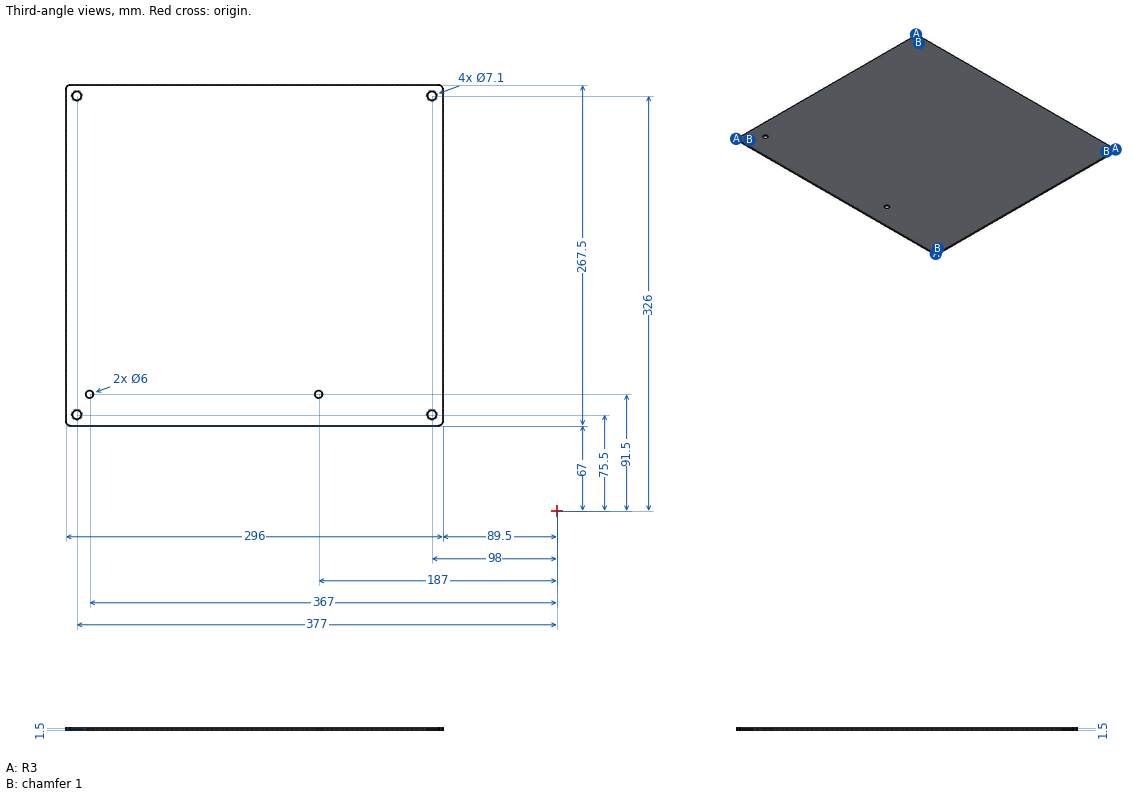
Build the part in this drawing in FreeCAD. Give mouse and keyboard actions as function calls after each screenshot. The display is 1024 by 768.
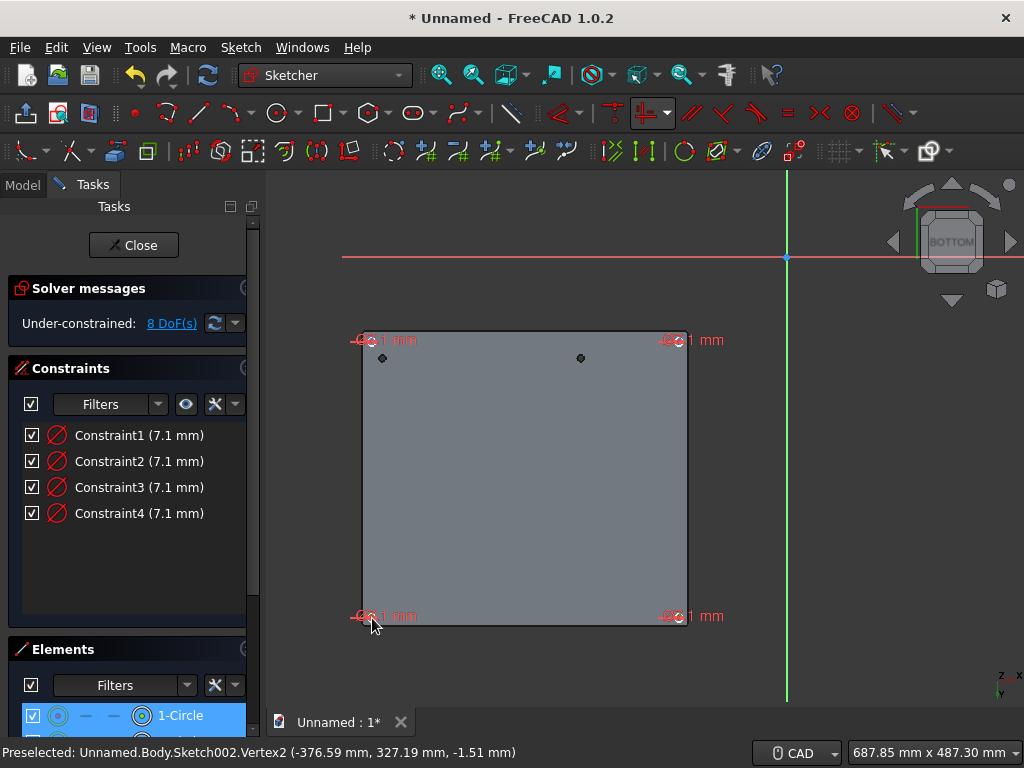
click(670, 114)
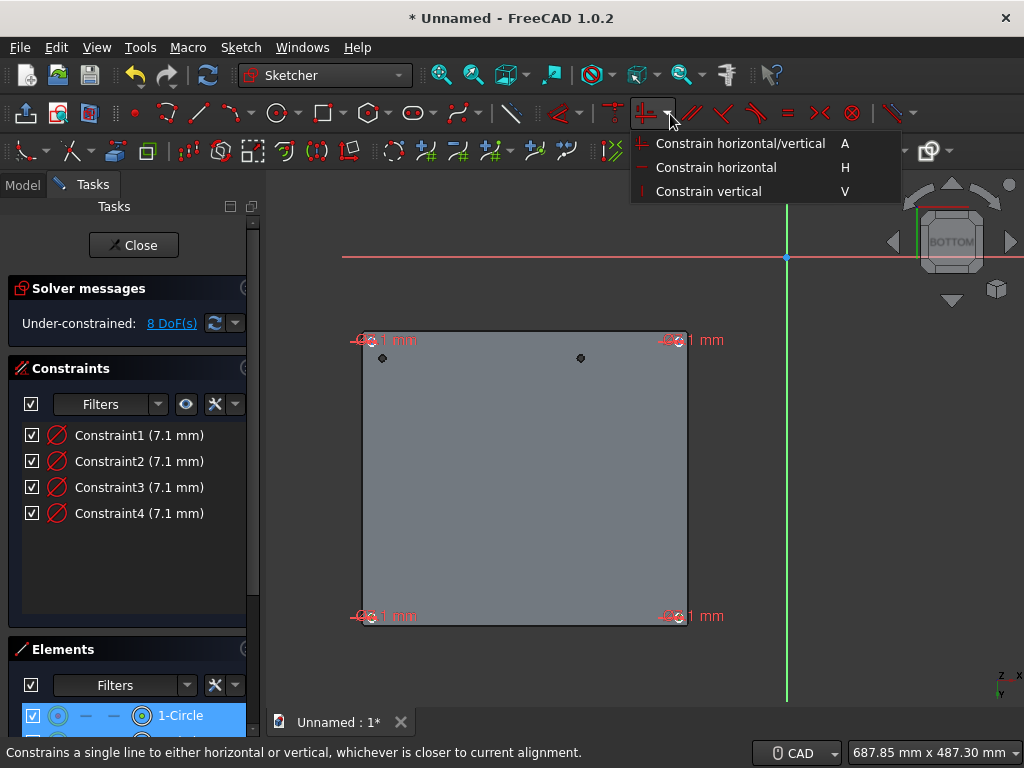
click(766, 167)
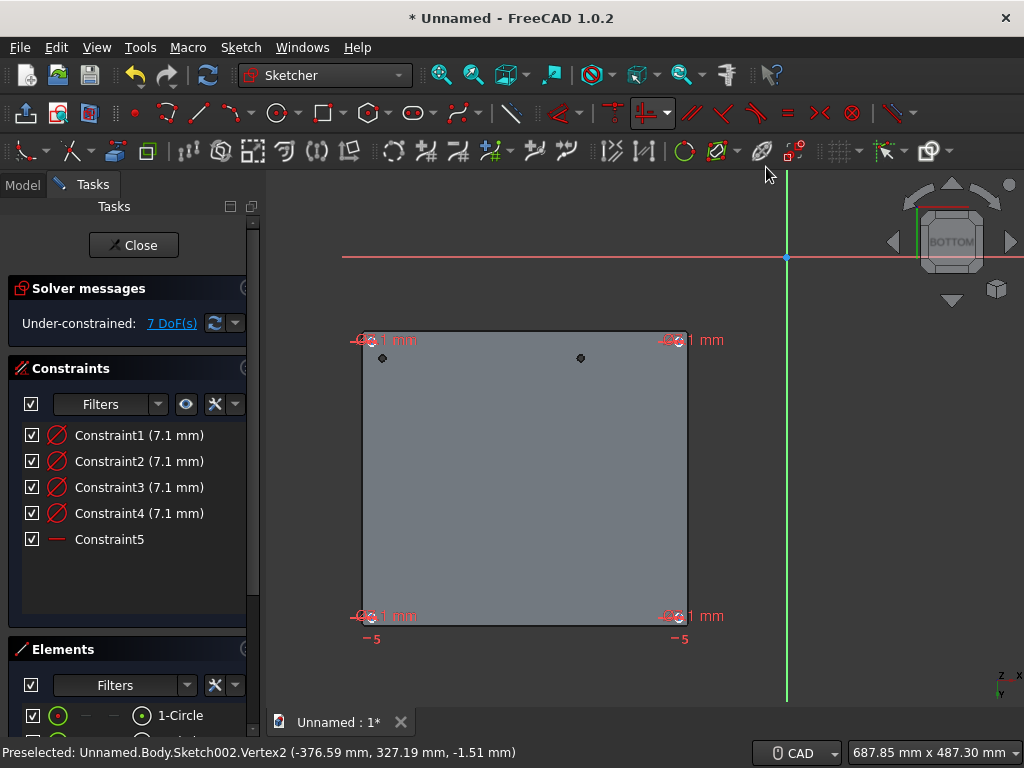
click(372, 618)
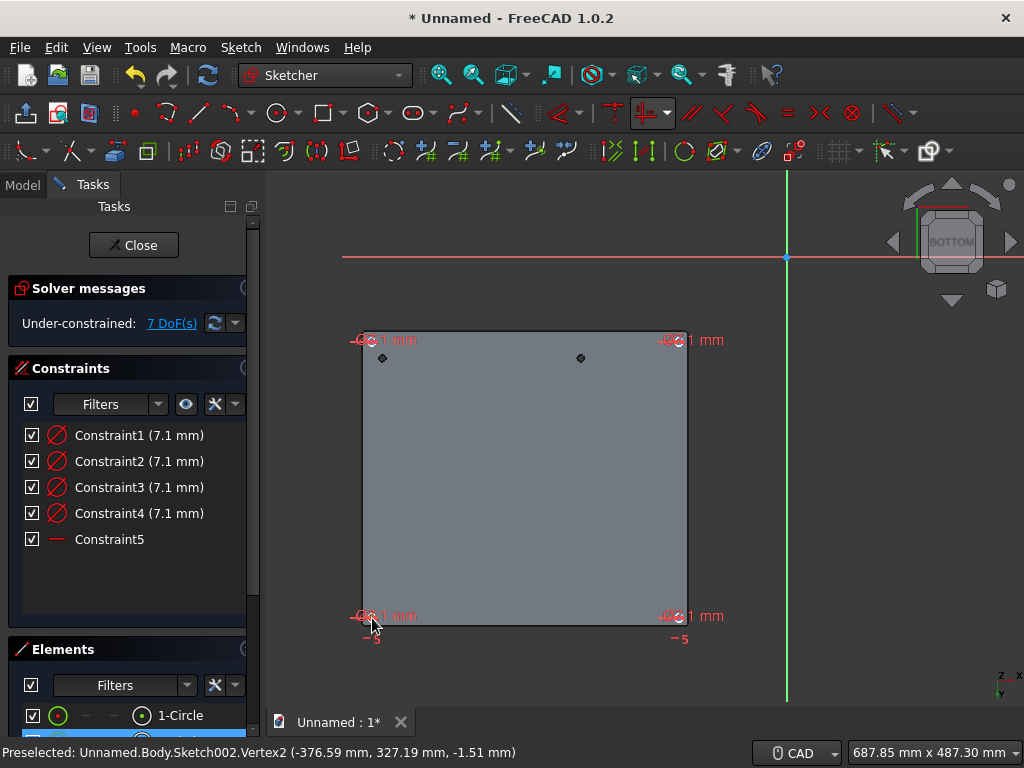
click(372, 342)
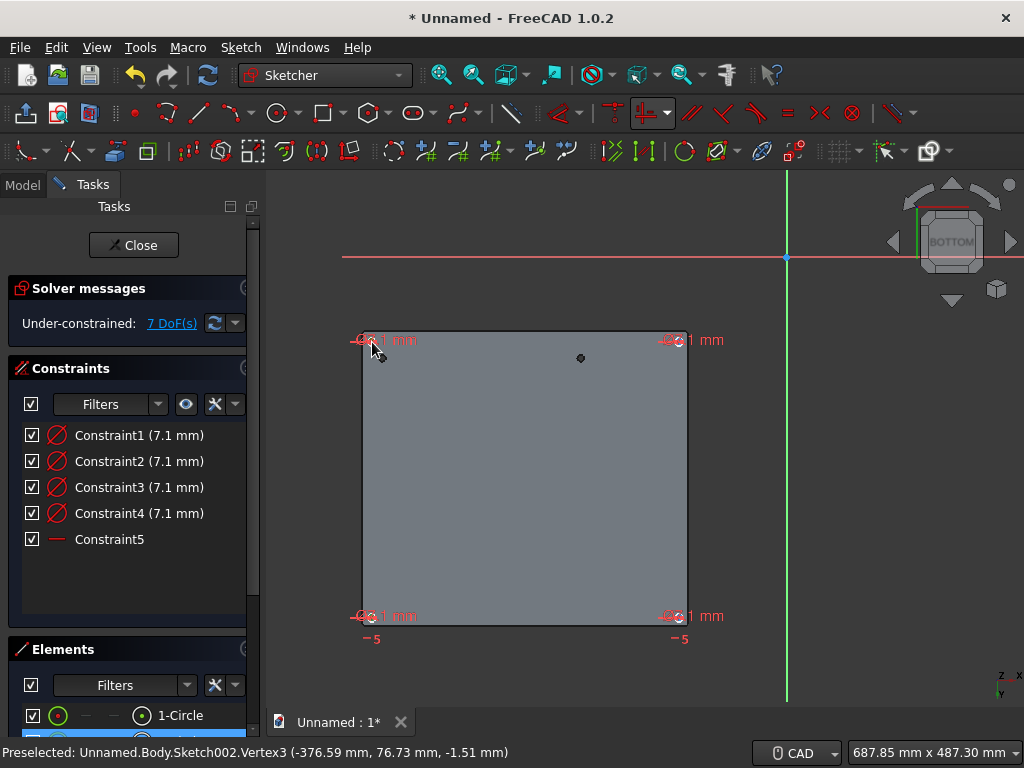
click(670, 114)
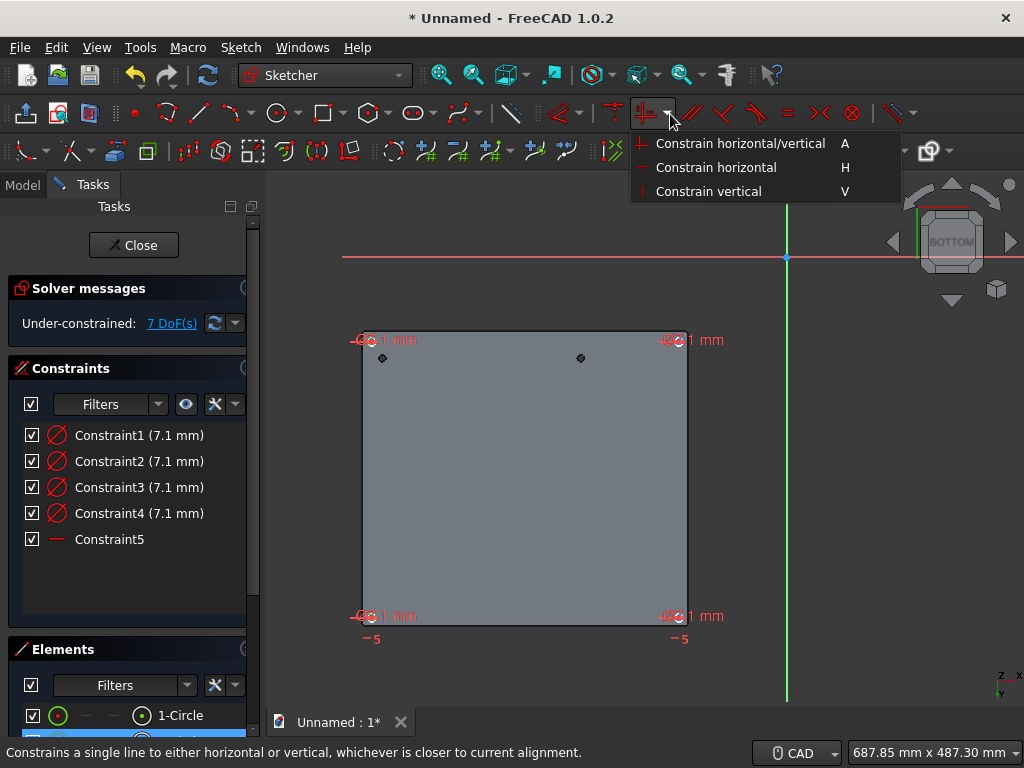
click(766, 191)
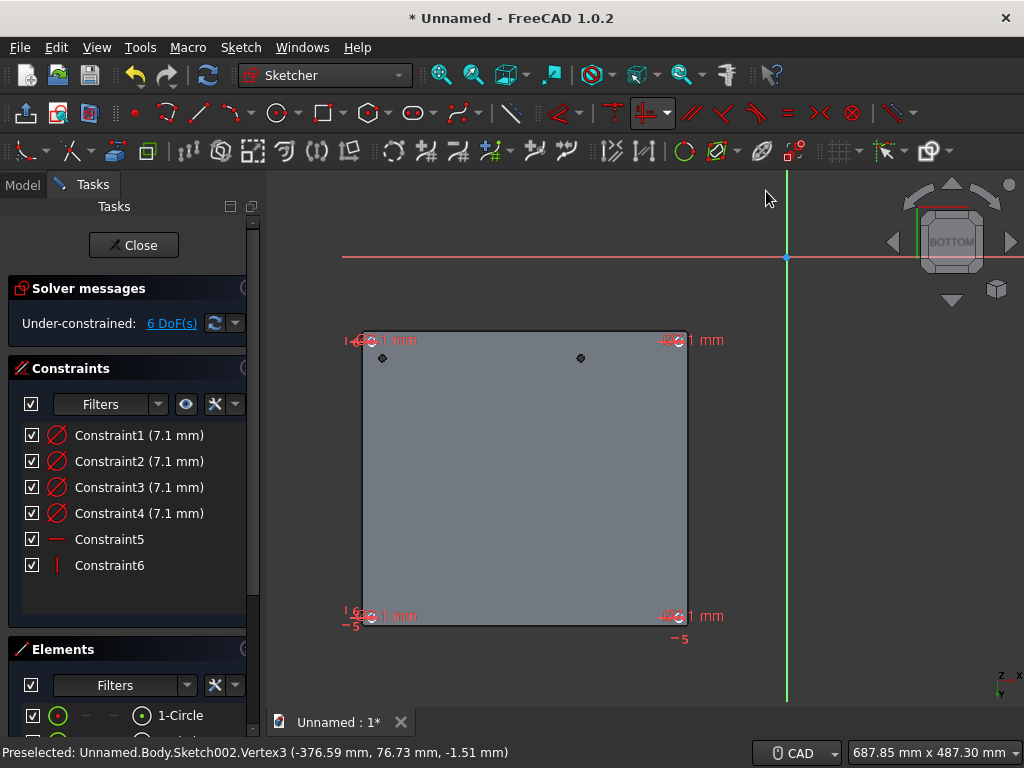
click(679, 618)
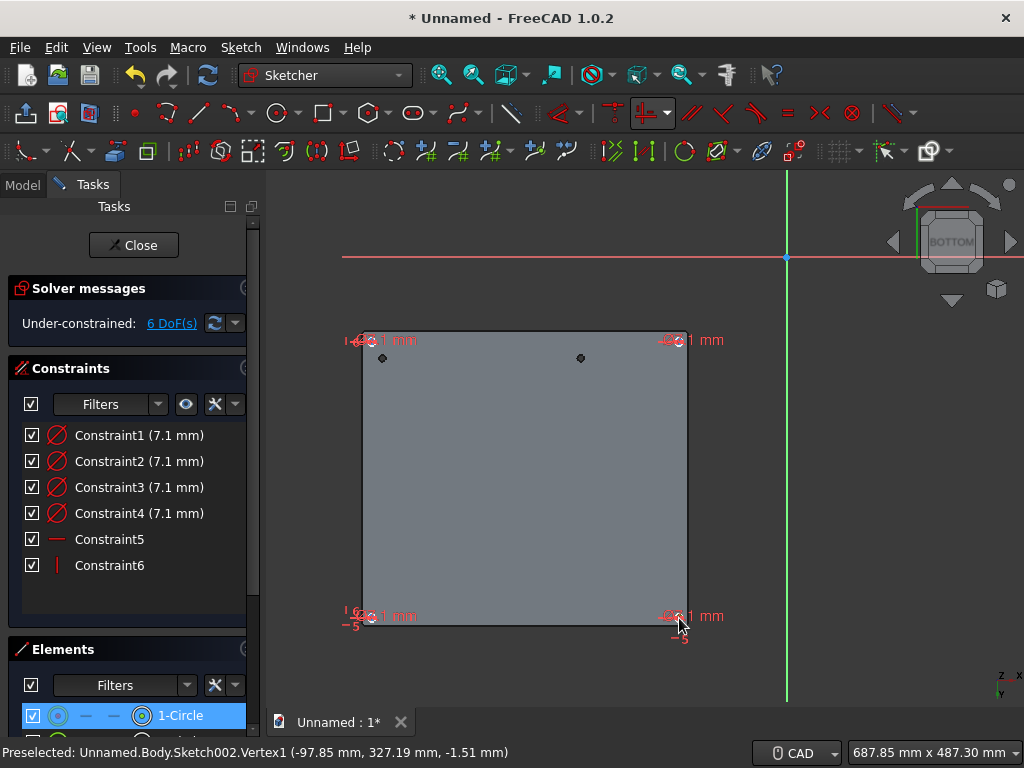
click(679, 342)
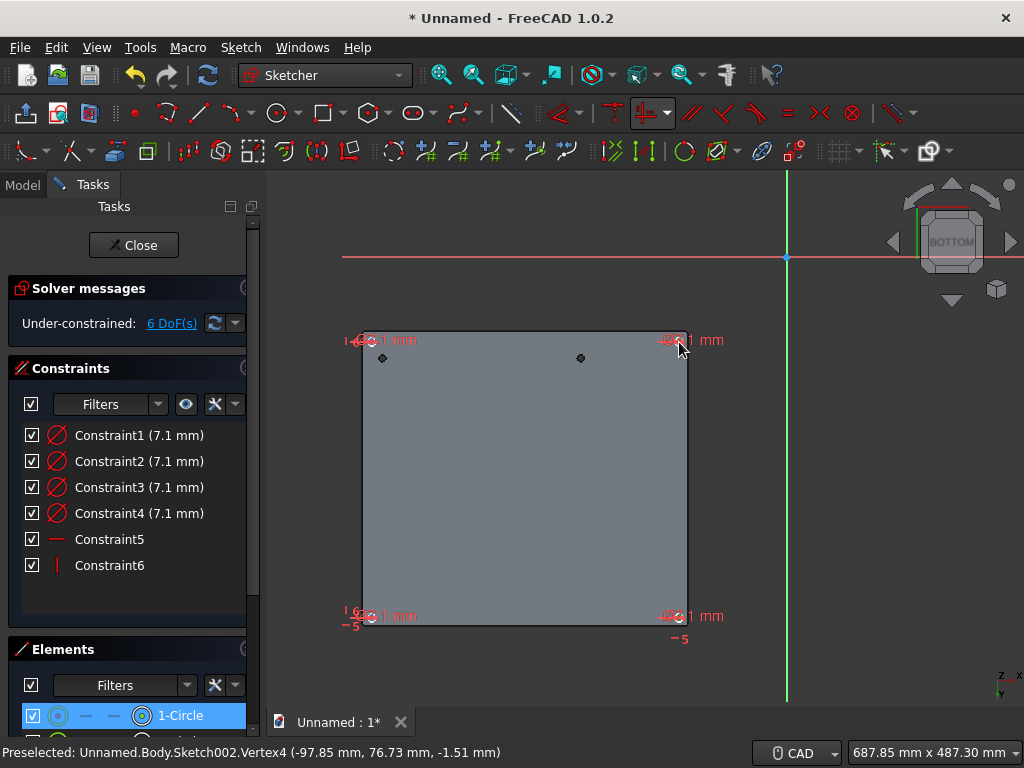
click(670, 114)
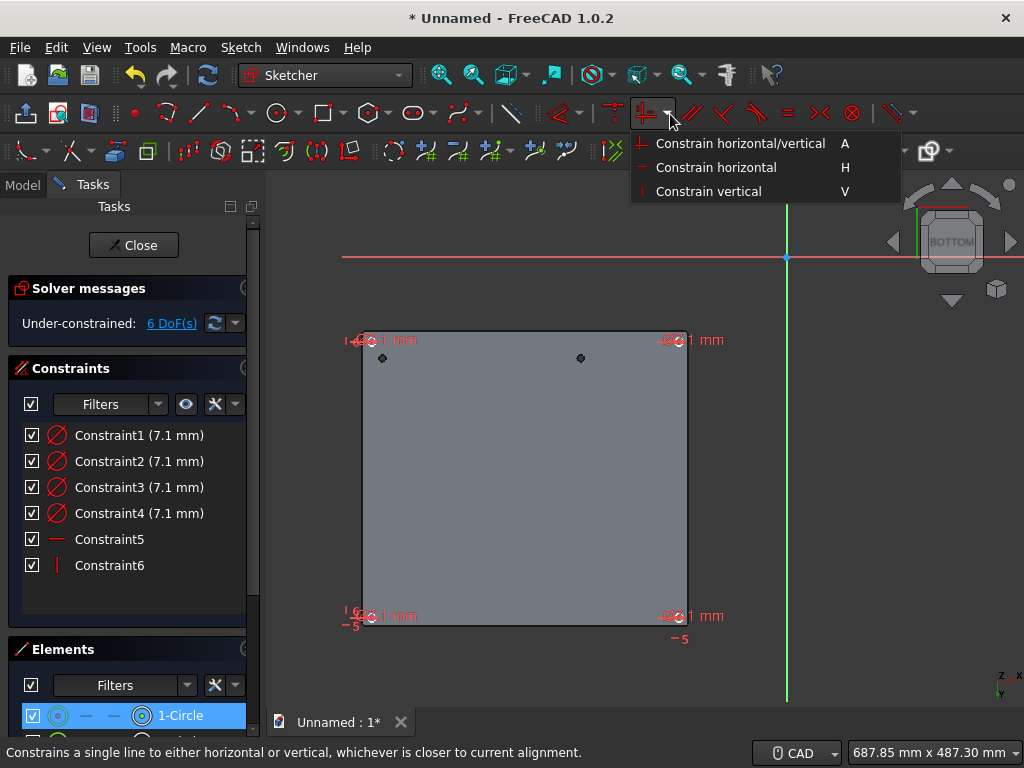
click(766, 191)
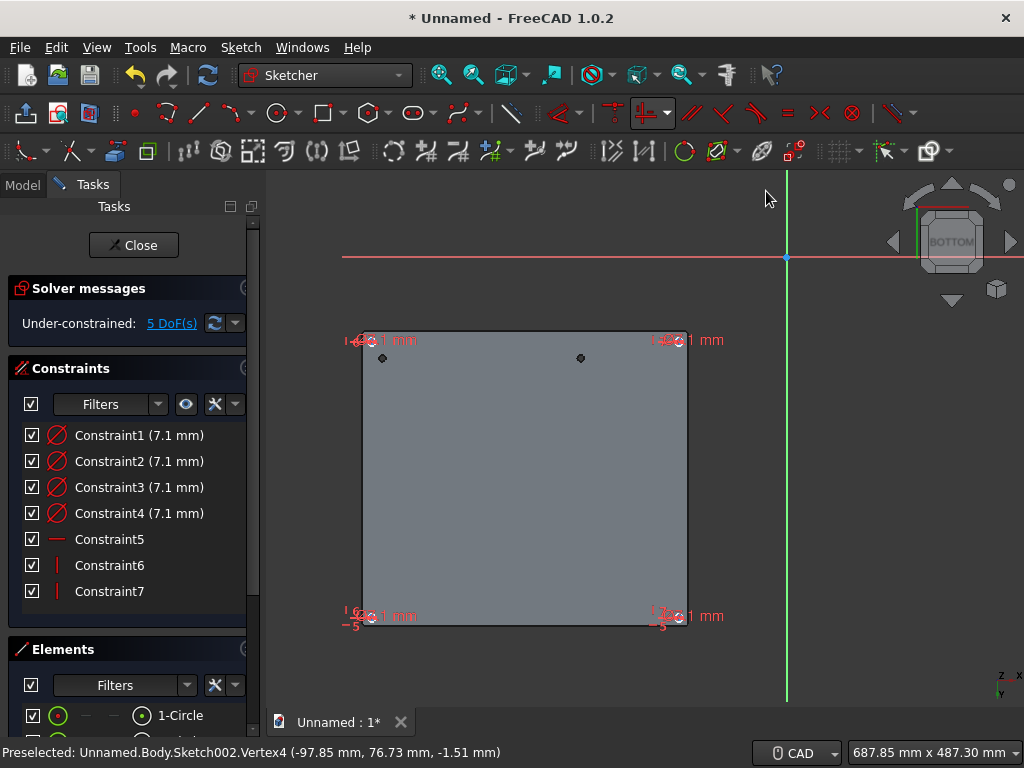
click(372, 342)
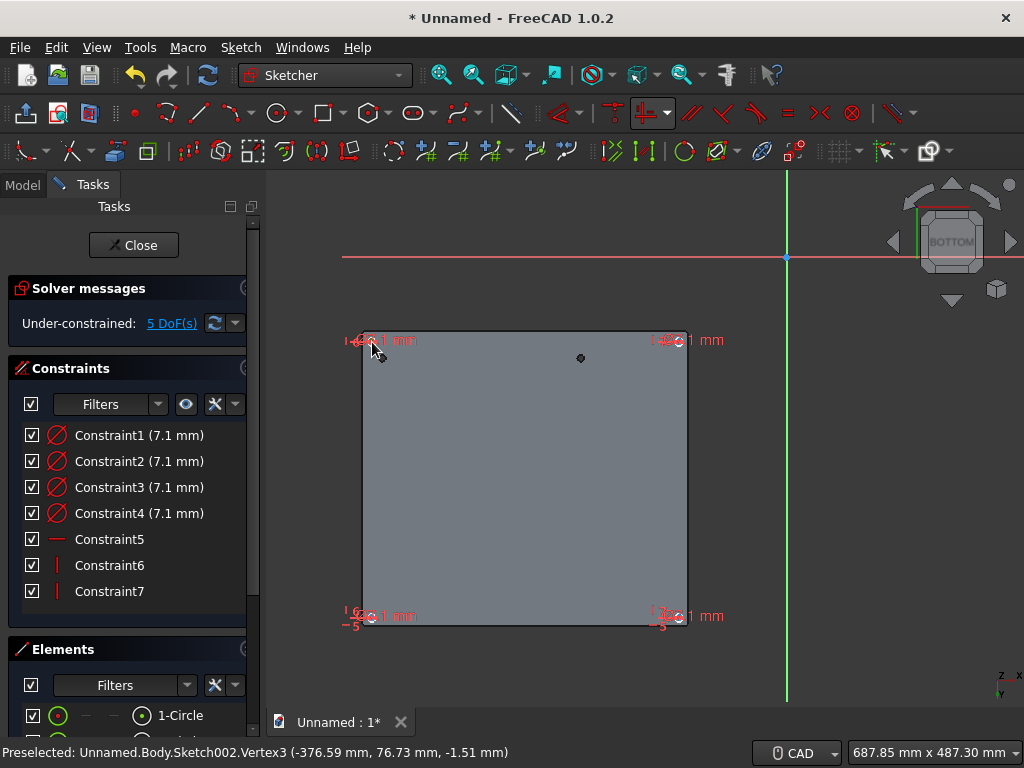
click(679, 342)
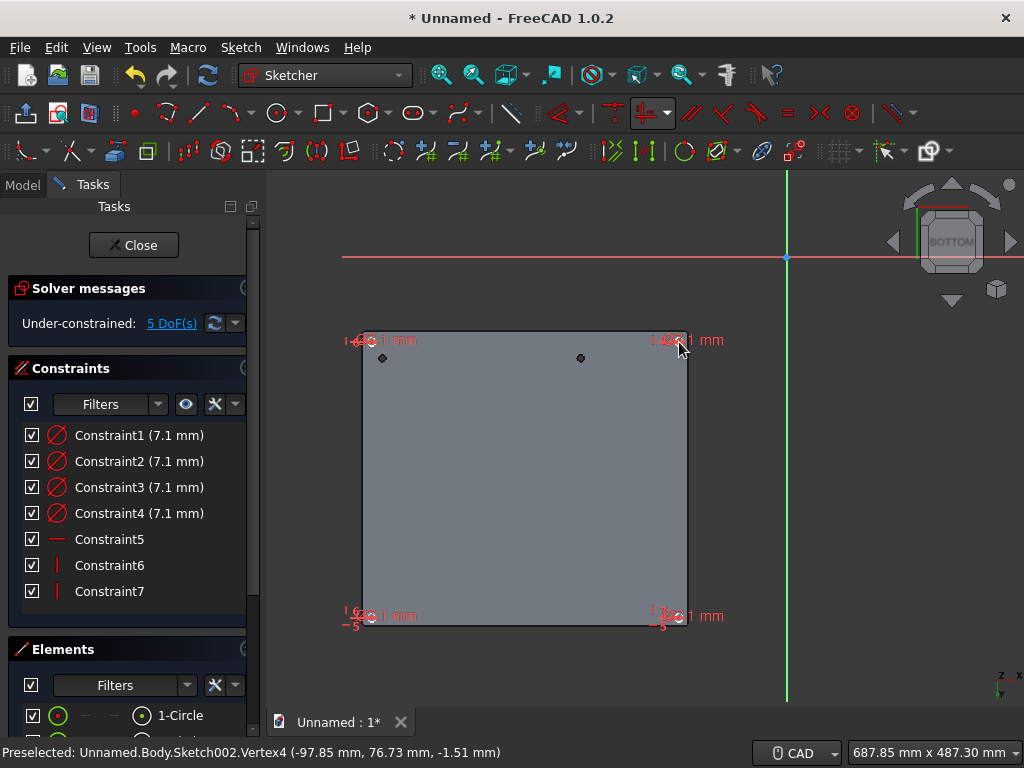
key(h)